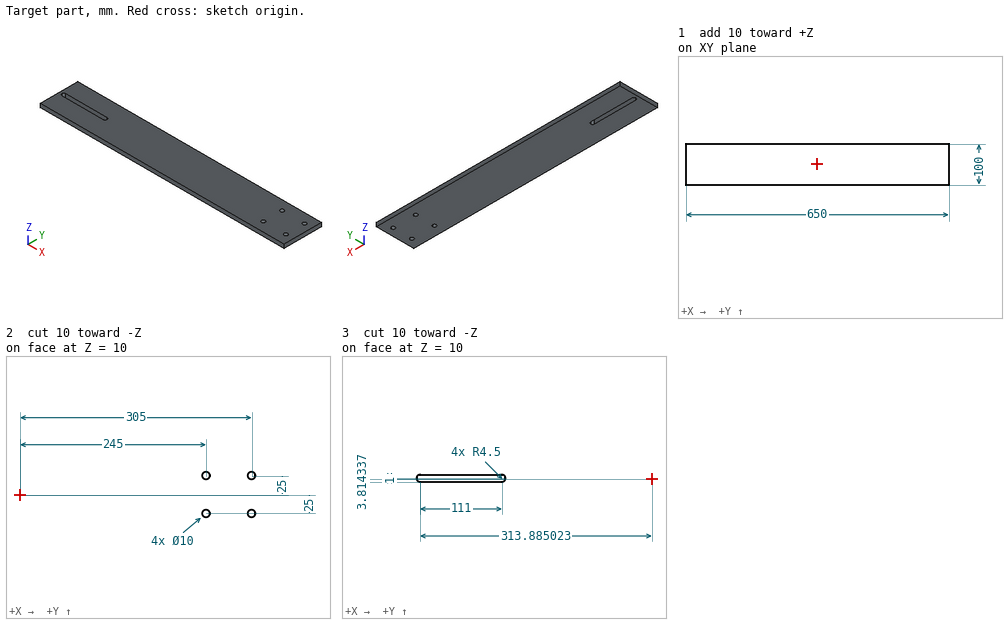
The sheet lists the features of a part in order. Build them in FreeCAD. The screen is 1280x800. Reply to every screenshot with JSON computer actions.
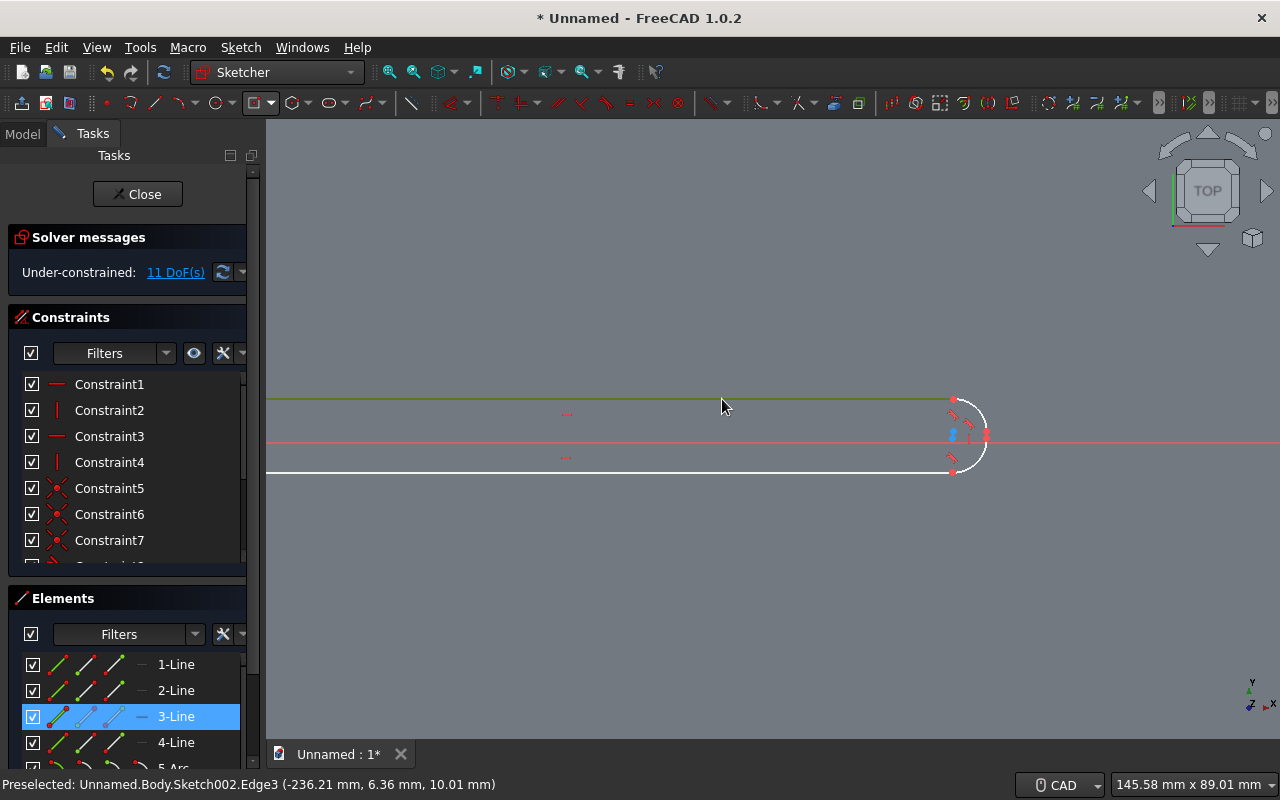
{"action": "scroll", "coordinate": [983, 417], "scroll_direction": "down", "scroll_amount": 2}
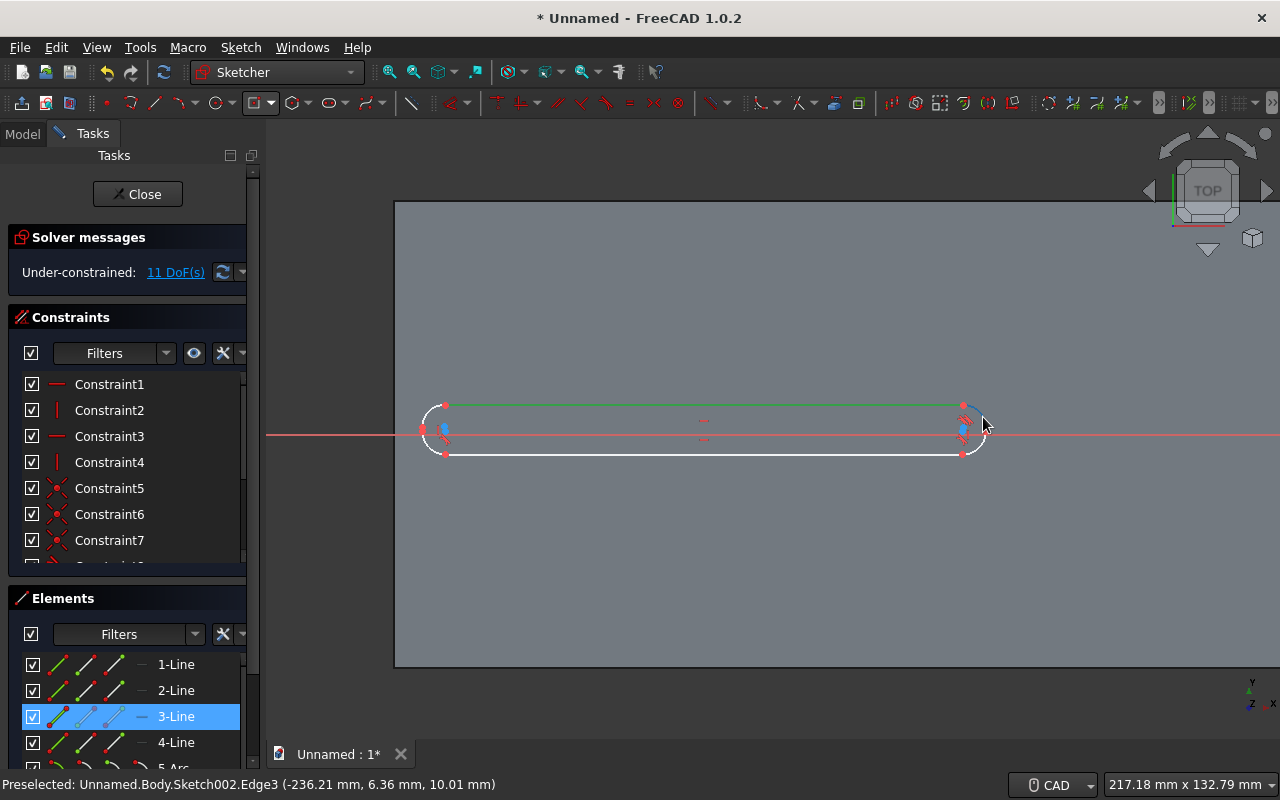
{"action": "scroll", "coordinate": [435, 407], "scroll_direction": "up", "scroll_amount": 2}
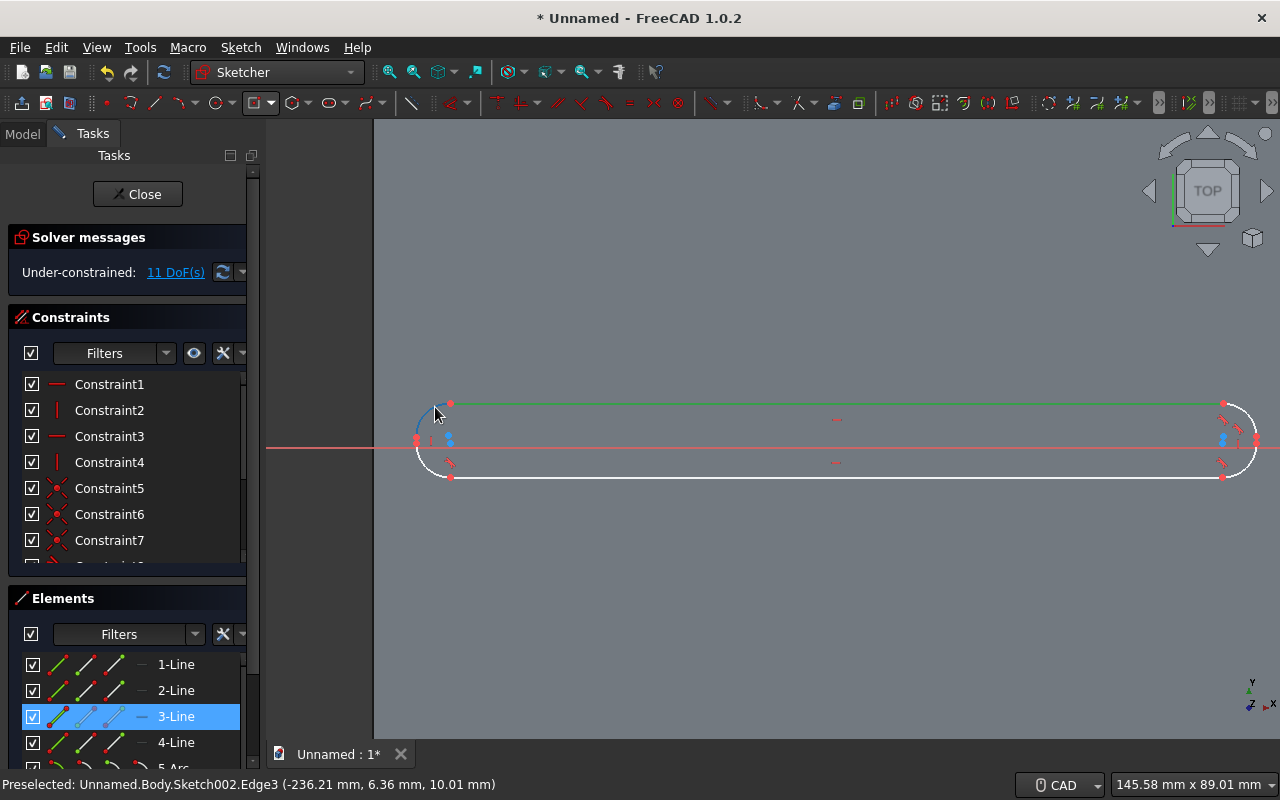
{"action": "left_click", "coordinate": [435, 407]}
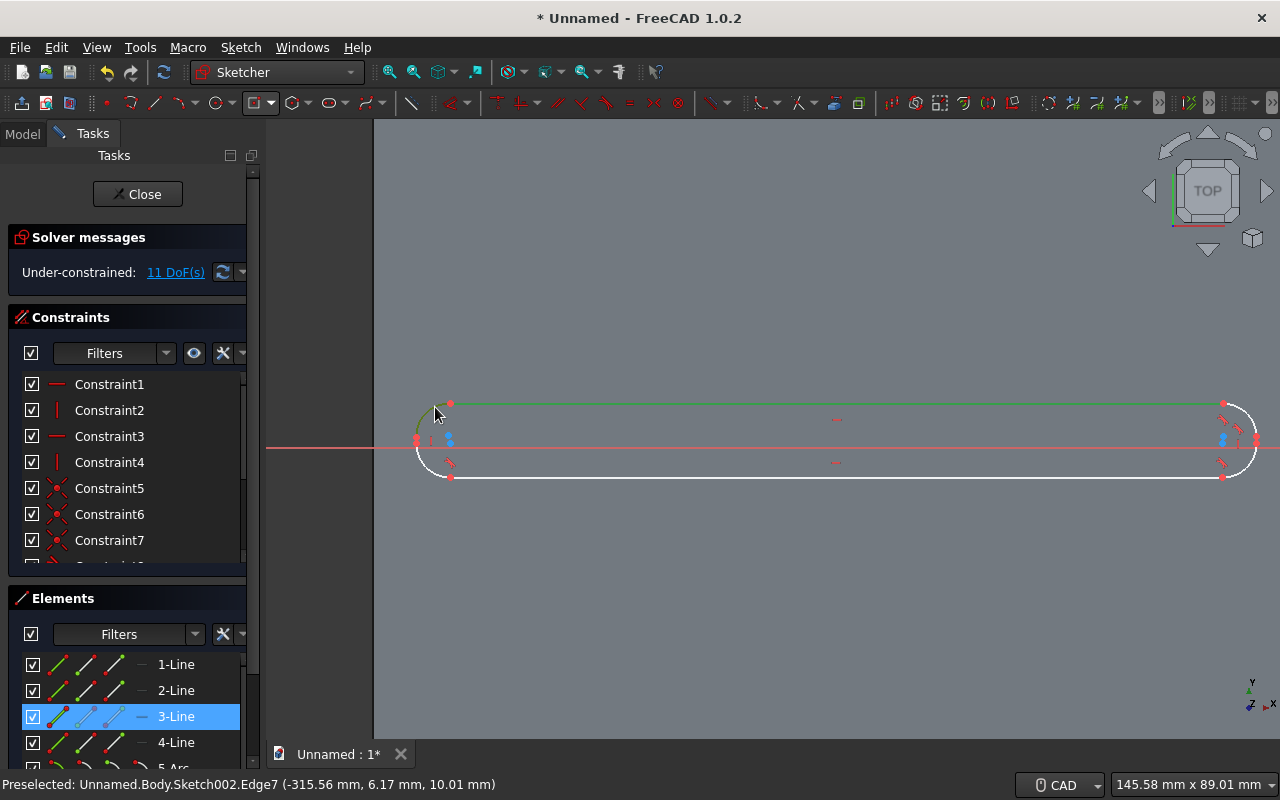
{"action": "key", "text": "t"}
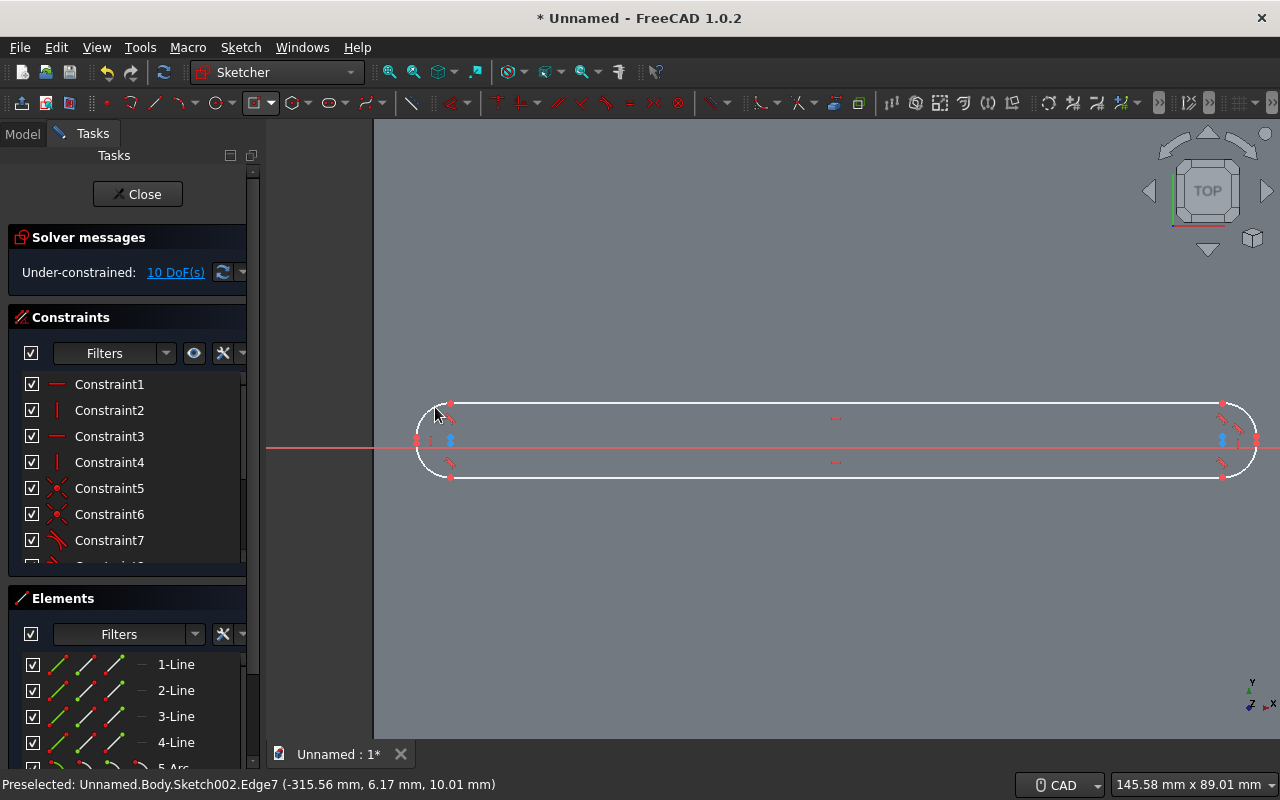
{"action": "scroll", "coordinate": [416, 440], "scroll_direction": "up", "scroll_amount": 8}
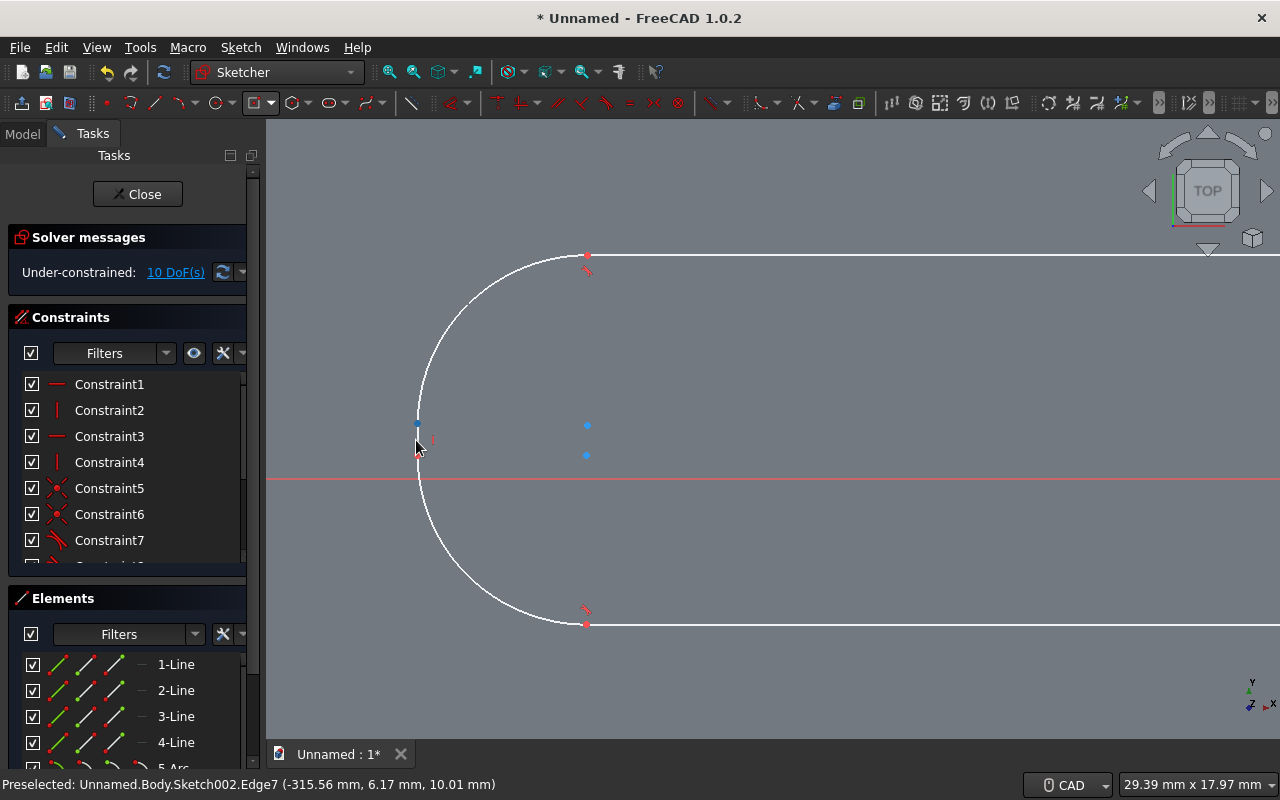
{"action": "left_click", "coordinate": [418, 440]}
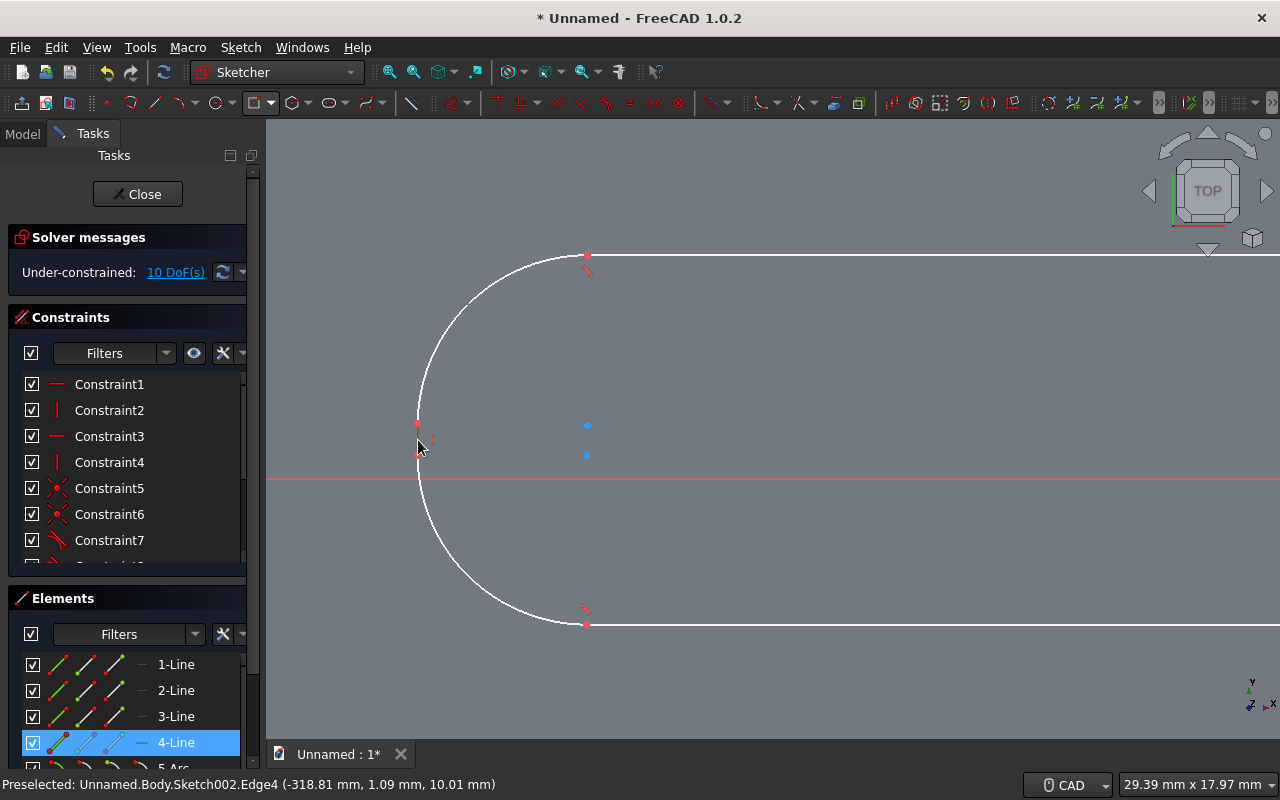
{"action": "scroll", "coordinate": [423, 428], "scroll_direction": "down", "scroll_amount": 10}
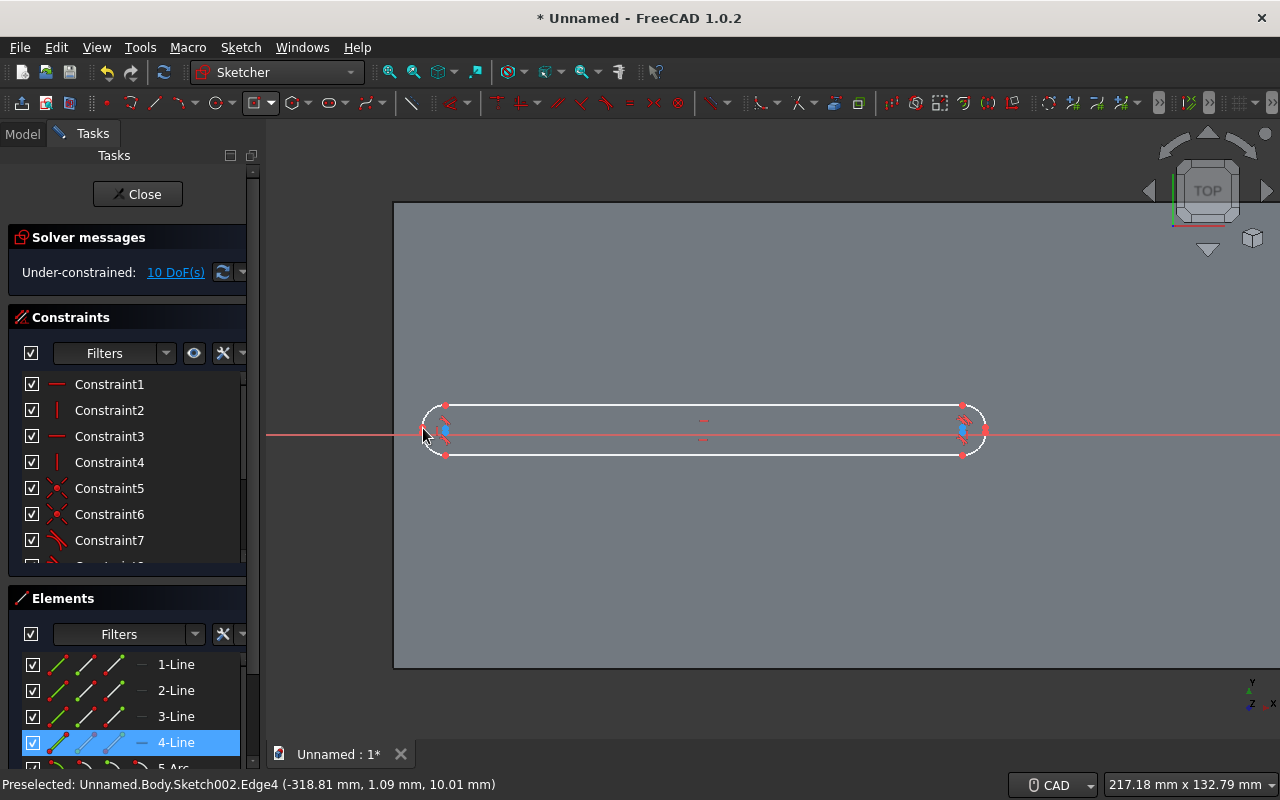
{"action": "scroll", "coordinate": [435, 408], "scroll_direction": "up", "scroll_amount": 2}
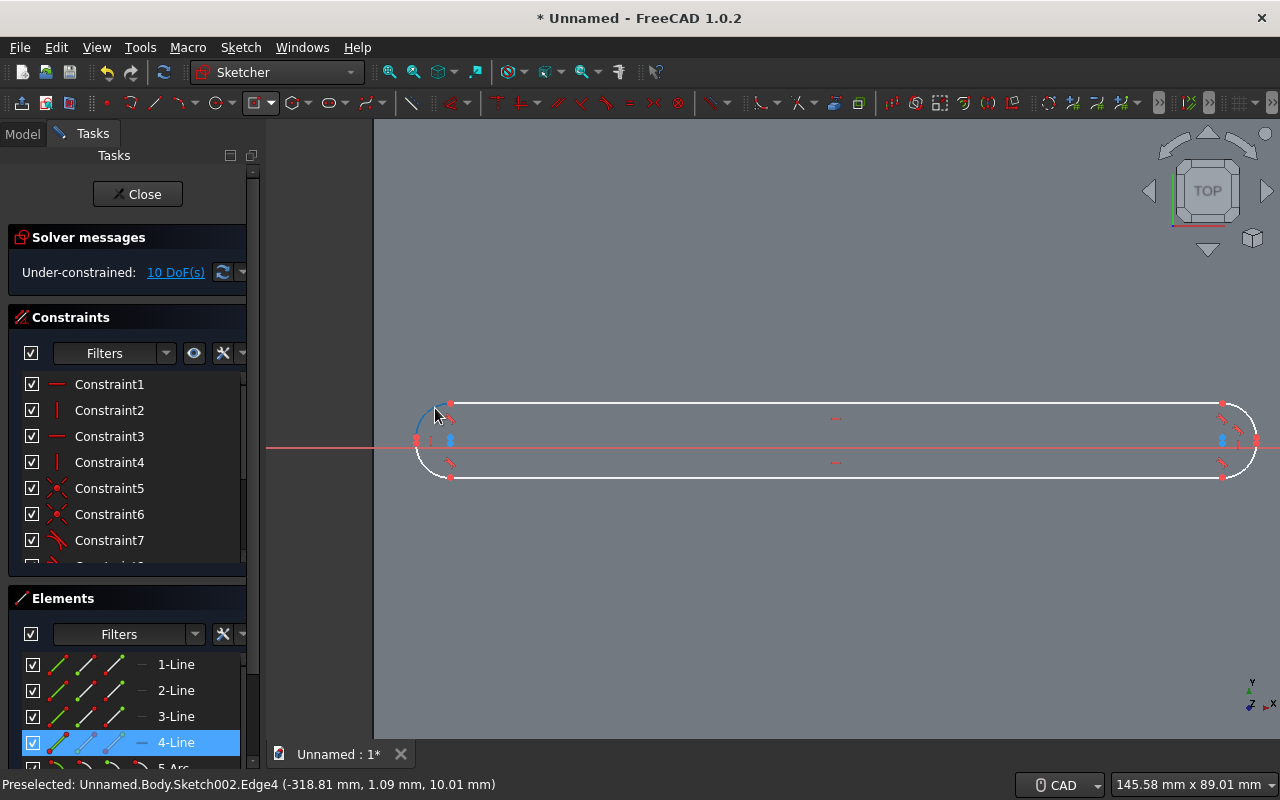
{"action": "left_click", "coordinate": [435, 407]}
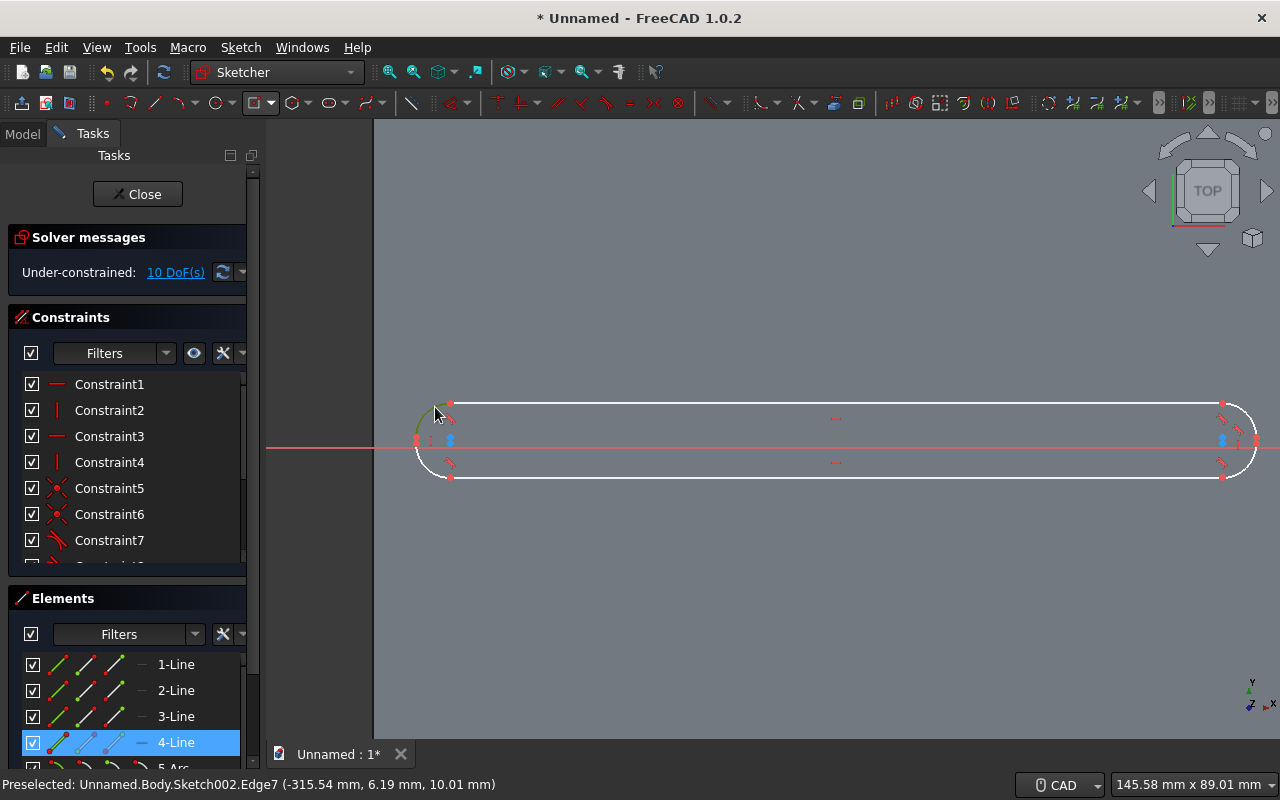
{"action": "key", "text": "t"}